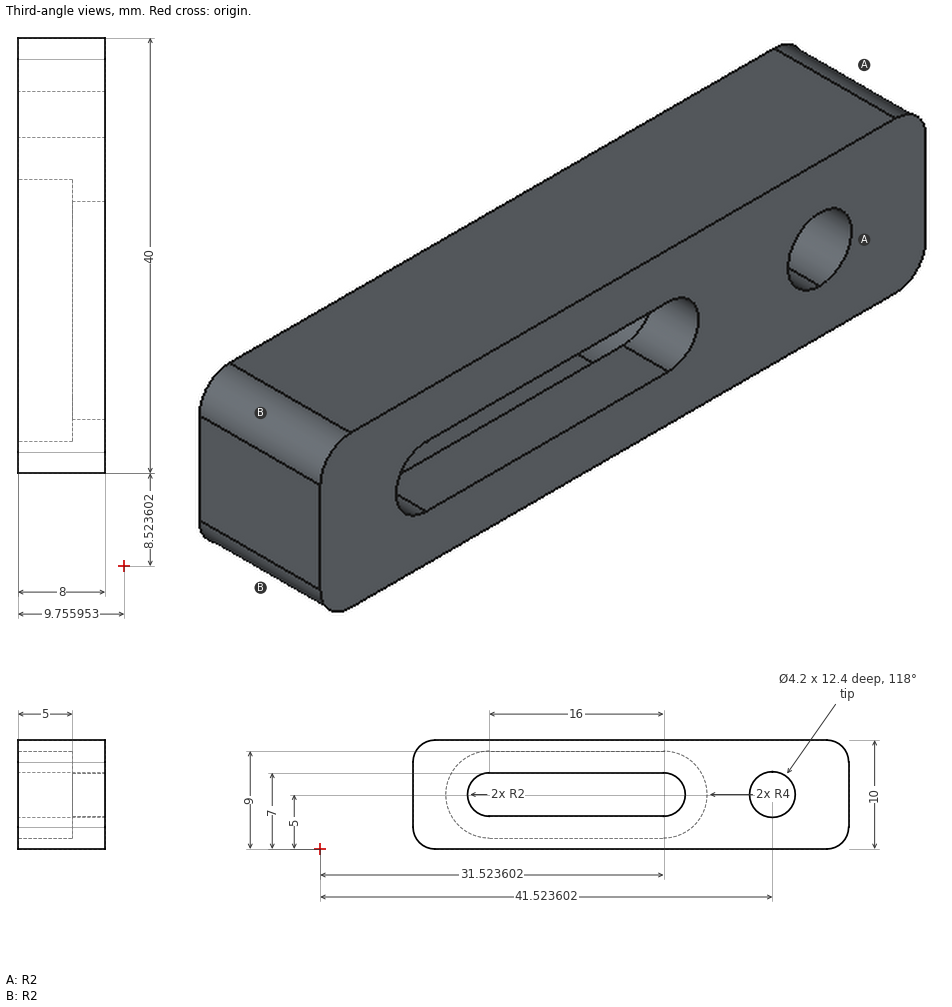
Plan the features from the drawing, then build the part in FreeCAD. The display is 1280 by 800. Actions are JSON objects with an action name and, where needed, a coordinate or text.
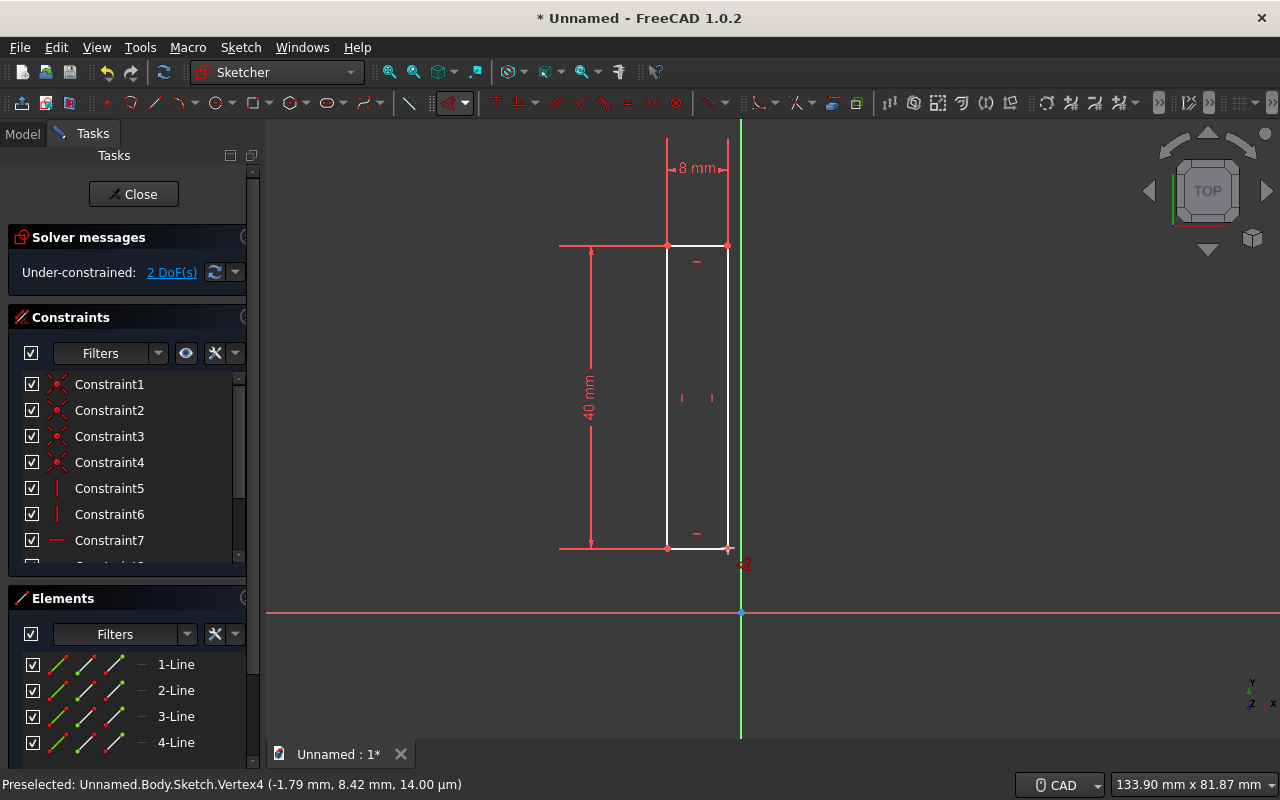
{"action": "left_click", "coordinate": [667, 246]}
{"action": "left_click", "coordinate": [704, 647]}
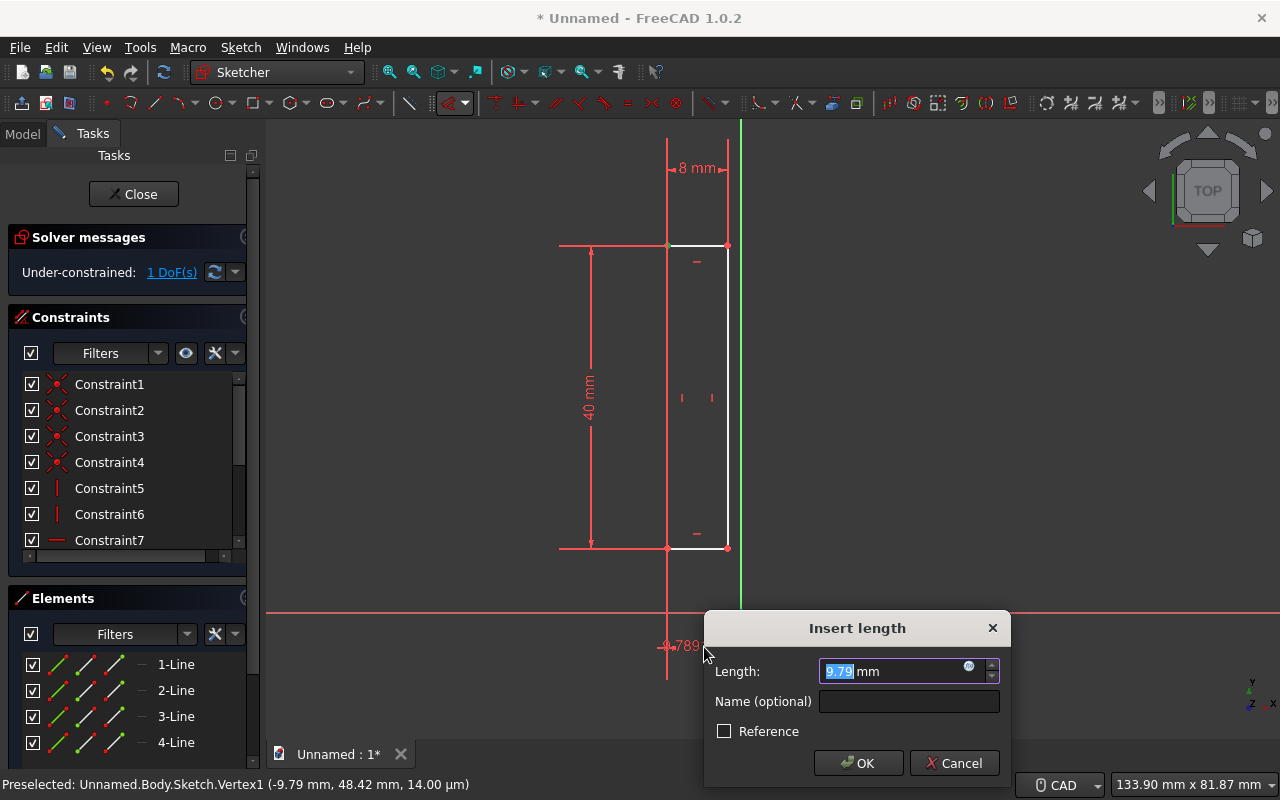
{"action": "type", "text": "9.755953"}
{"action": "key", "text": "Return"}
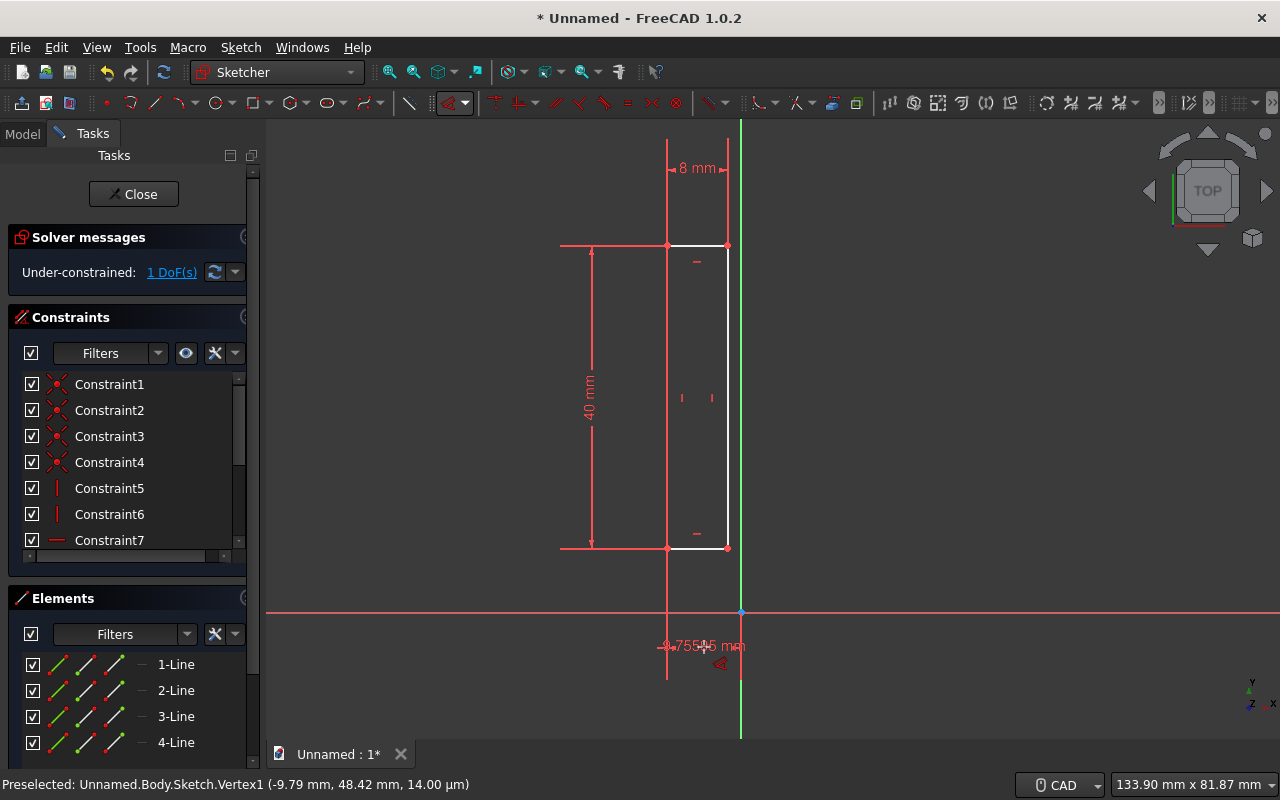
{"action": "left_click", "coordinate": [667, 549]}
{"action": "left_click", "coordinate": [633, 581]}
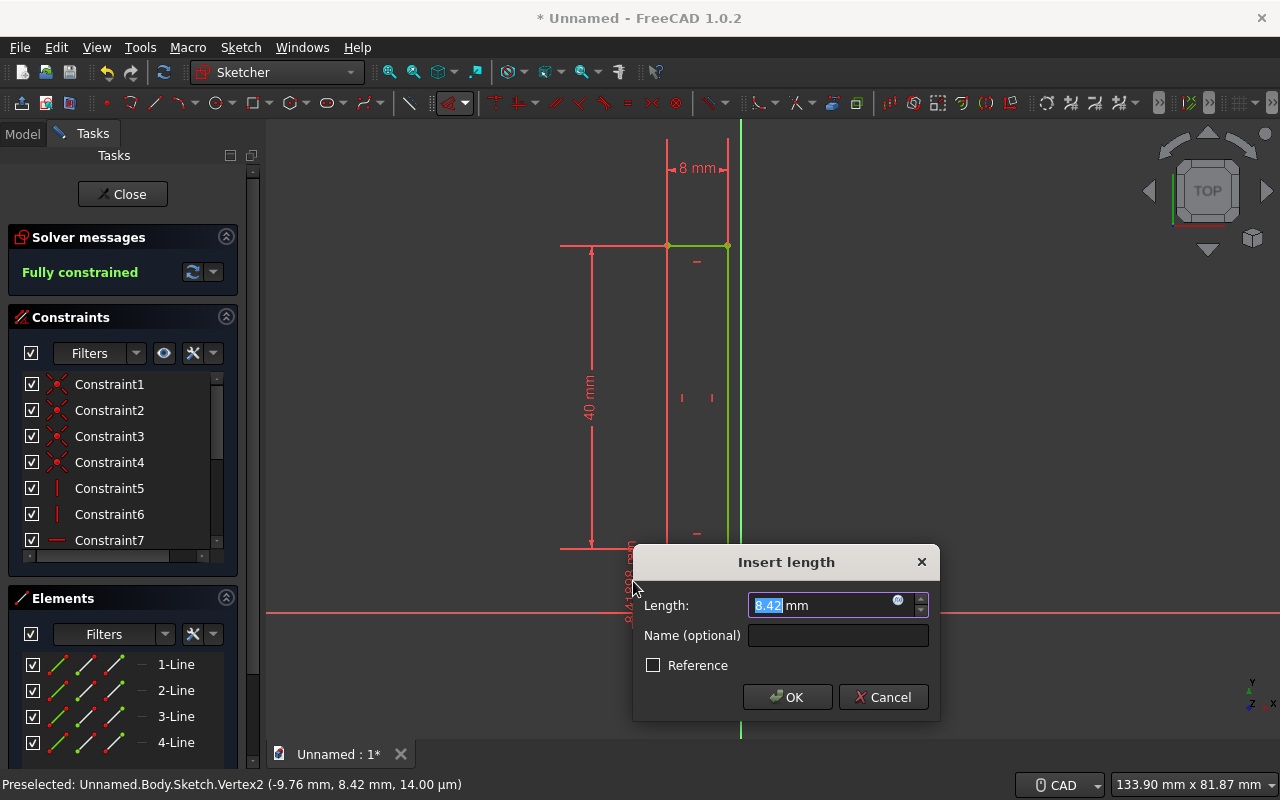
{"action": "type", "text": "8.523602"}
{"action": "key", "text": "Return"}
{"action": "key", "text": "Escape"}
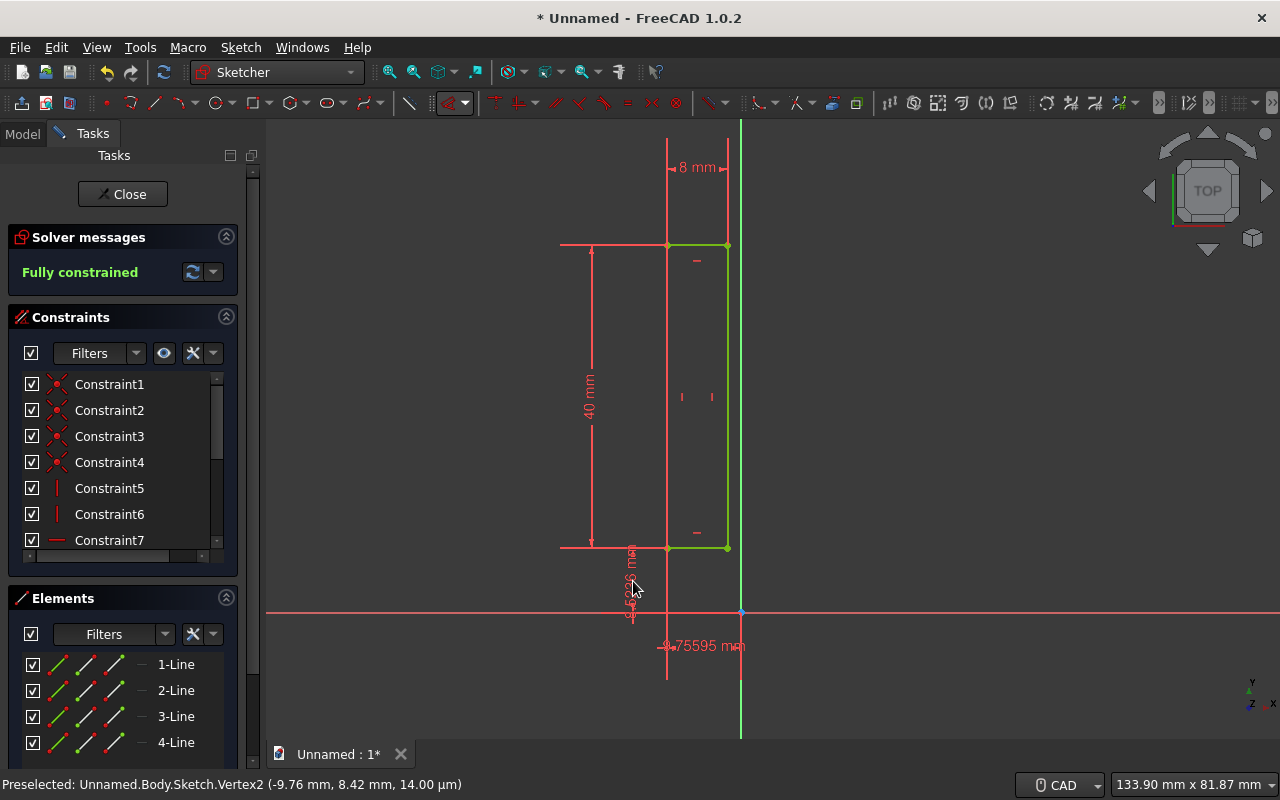
{"action": "left_click", "coordinate": [123, 194]}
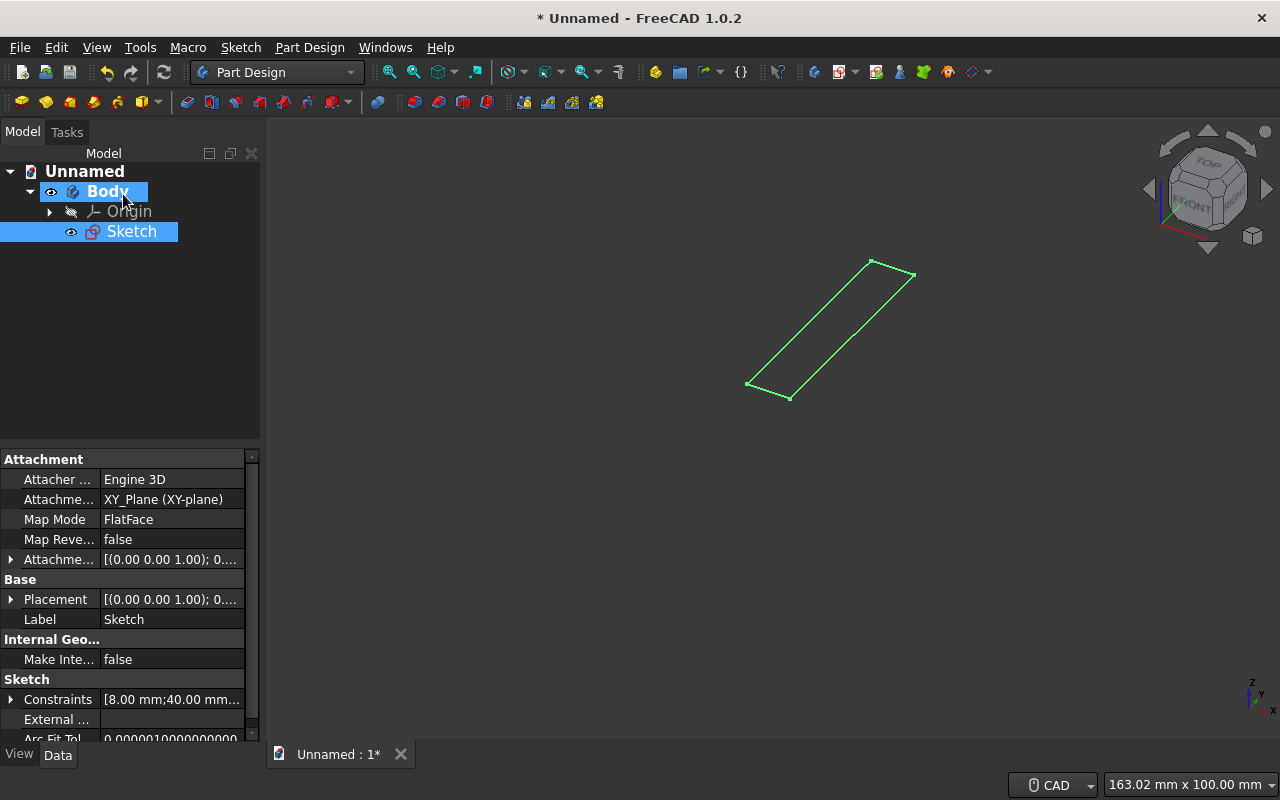
{"action": "left_click", "coordinate": [22, 102]}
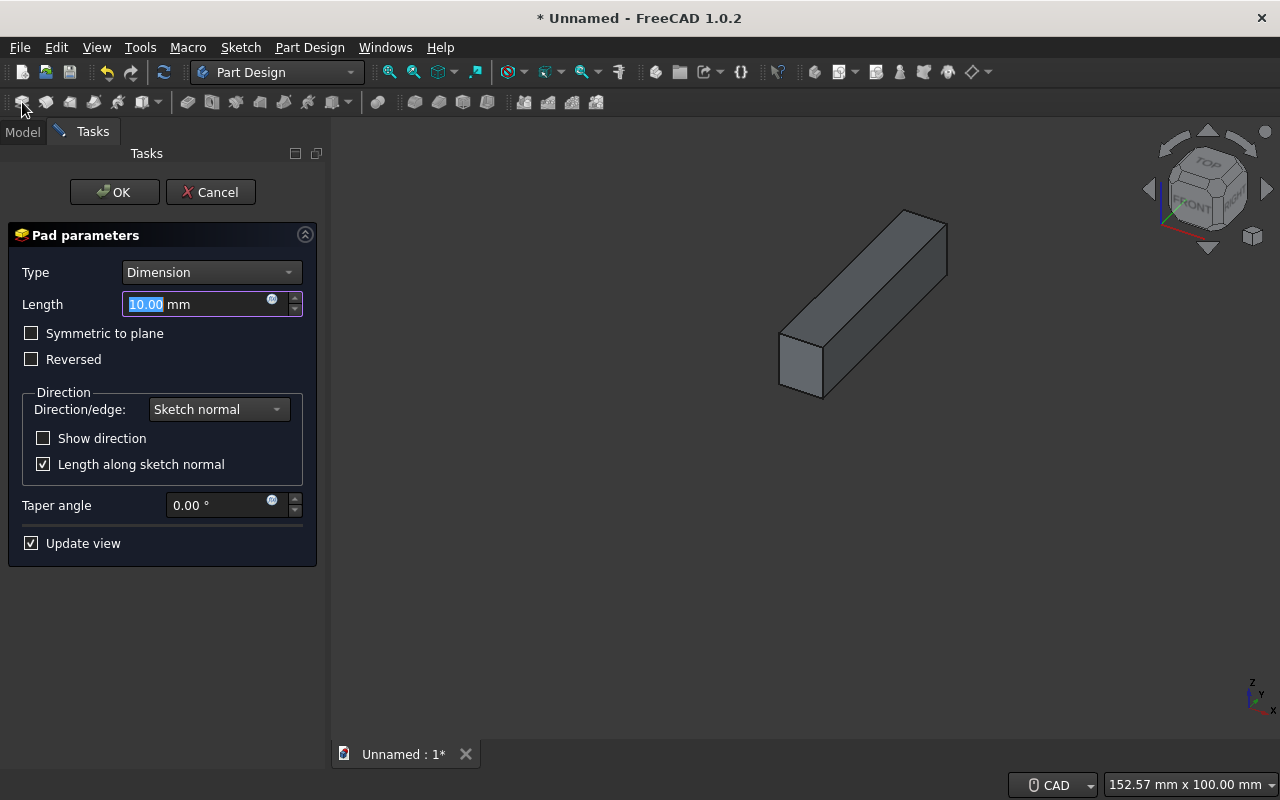
{"action": "type", "text": "10"}
{"action": "key", "text": "Tab"}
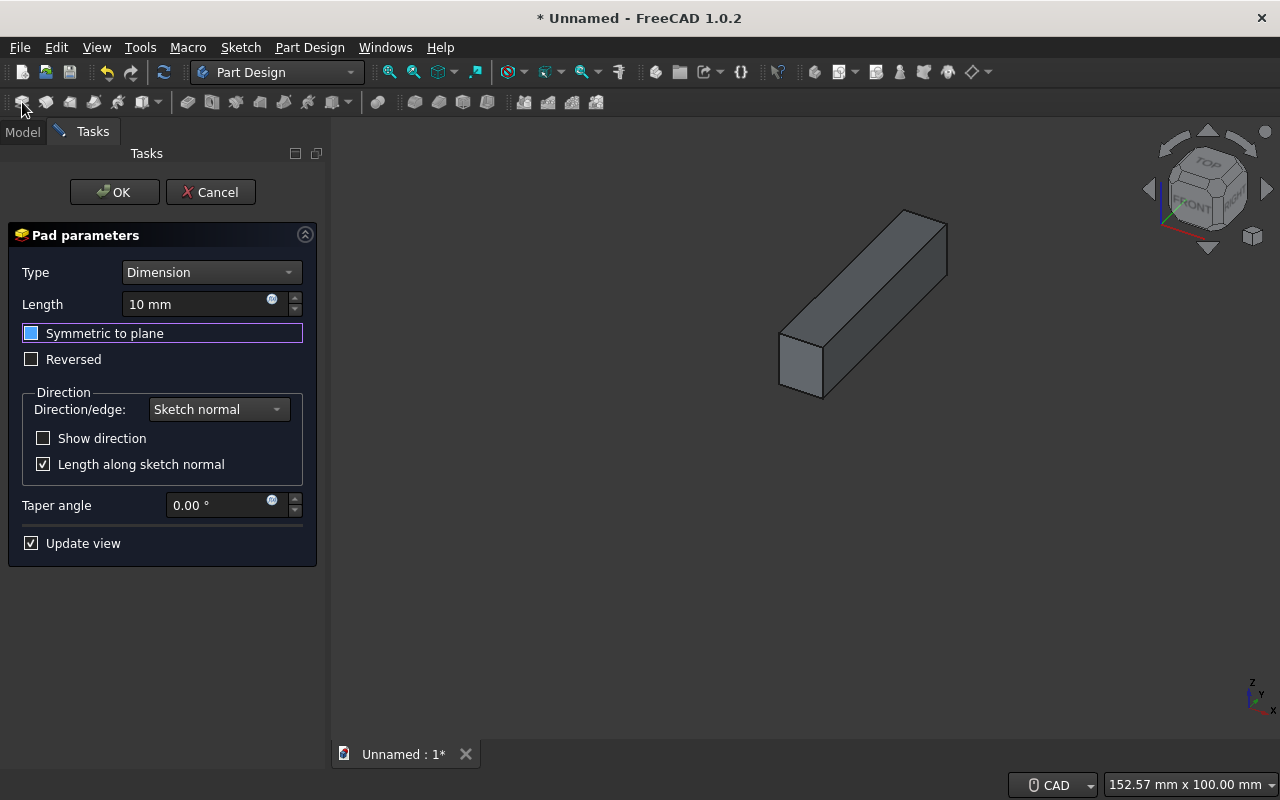
{"action": "left_click", "coordinate": [115, 192]}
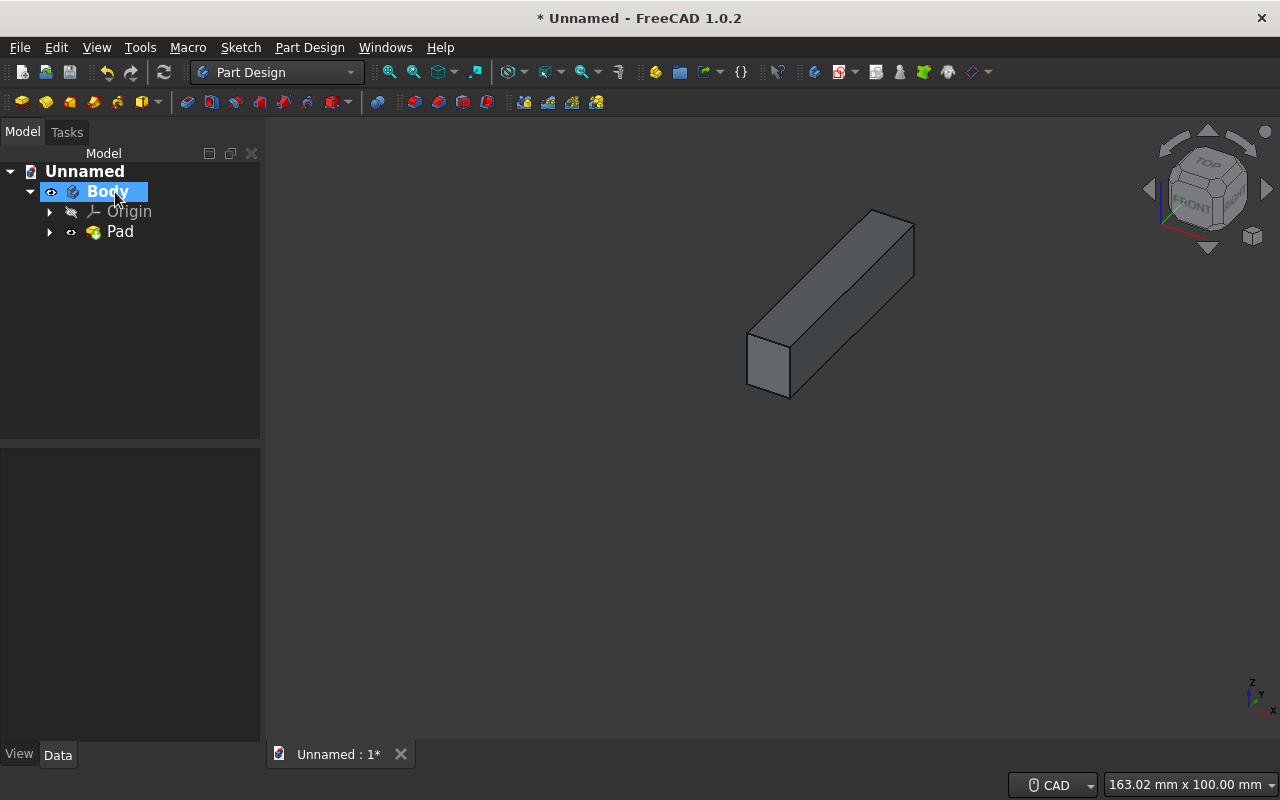
{"action": "key", "text": "v f"}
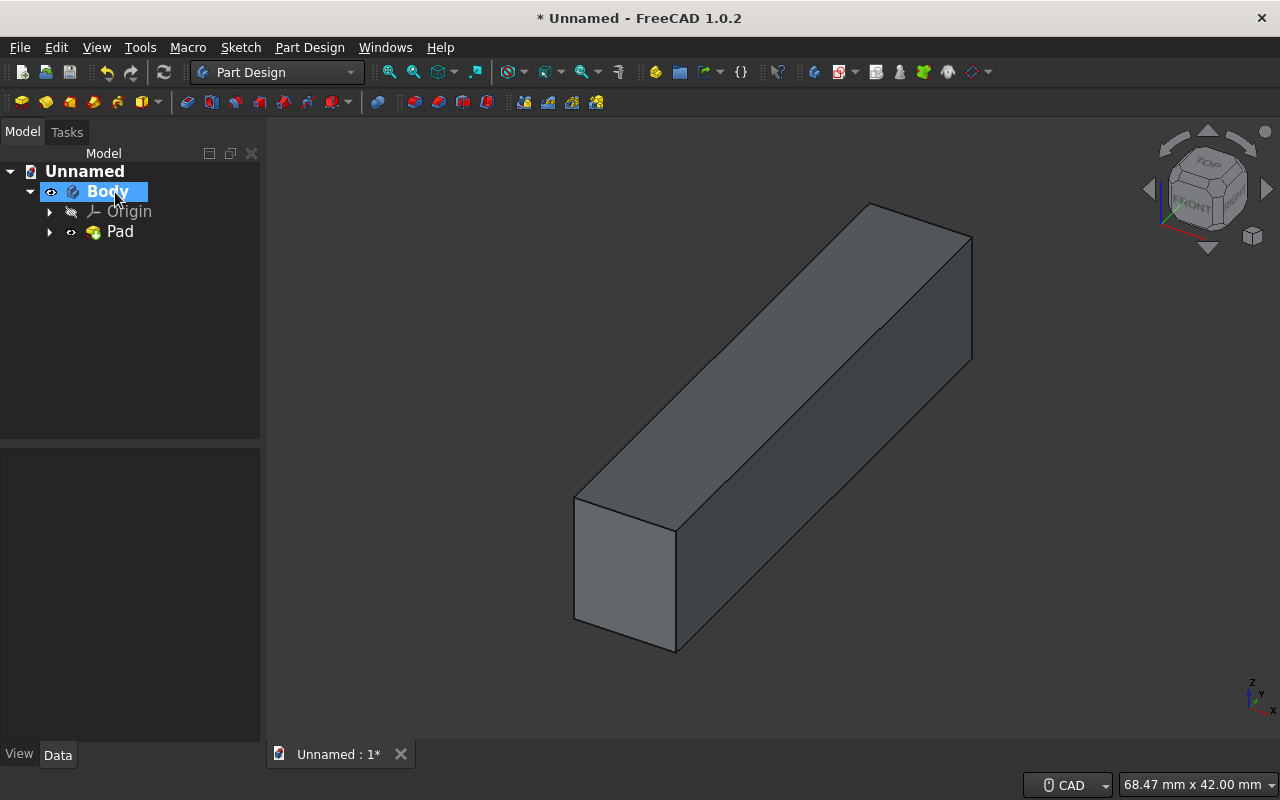
{"action": "left_click", "coordinate": [909, 360]}